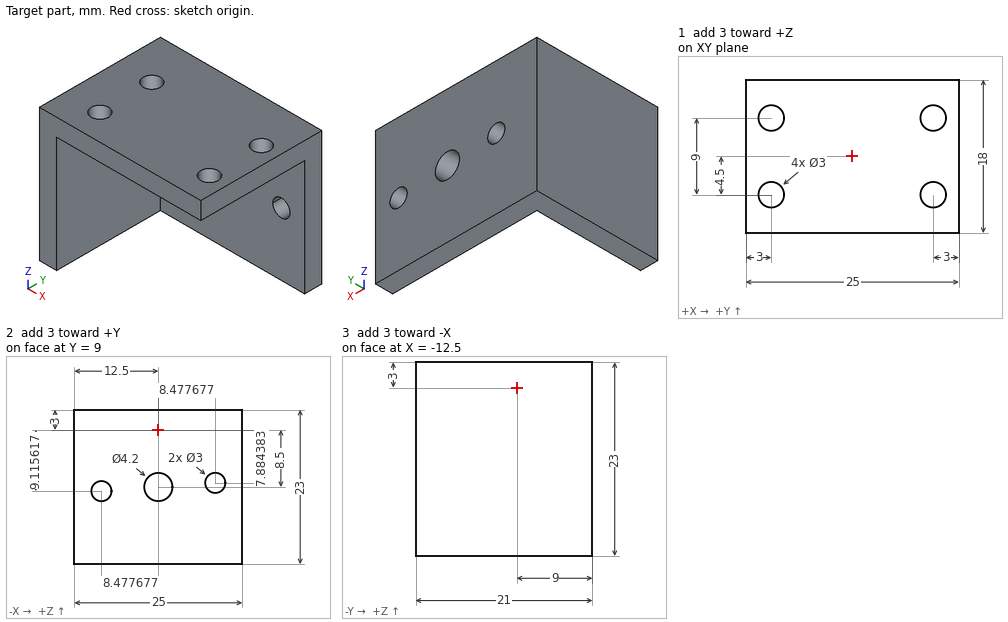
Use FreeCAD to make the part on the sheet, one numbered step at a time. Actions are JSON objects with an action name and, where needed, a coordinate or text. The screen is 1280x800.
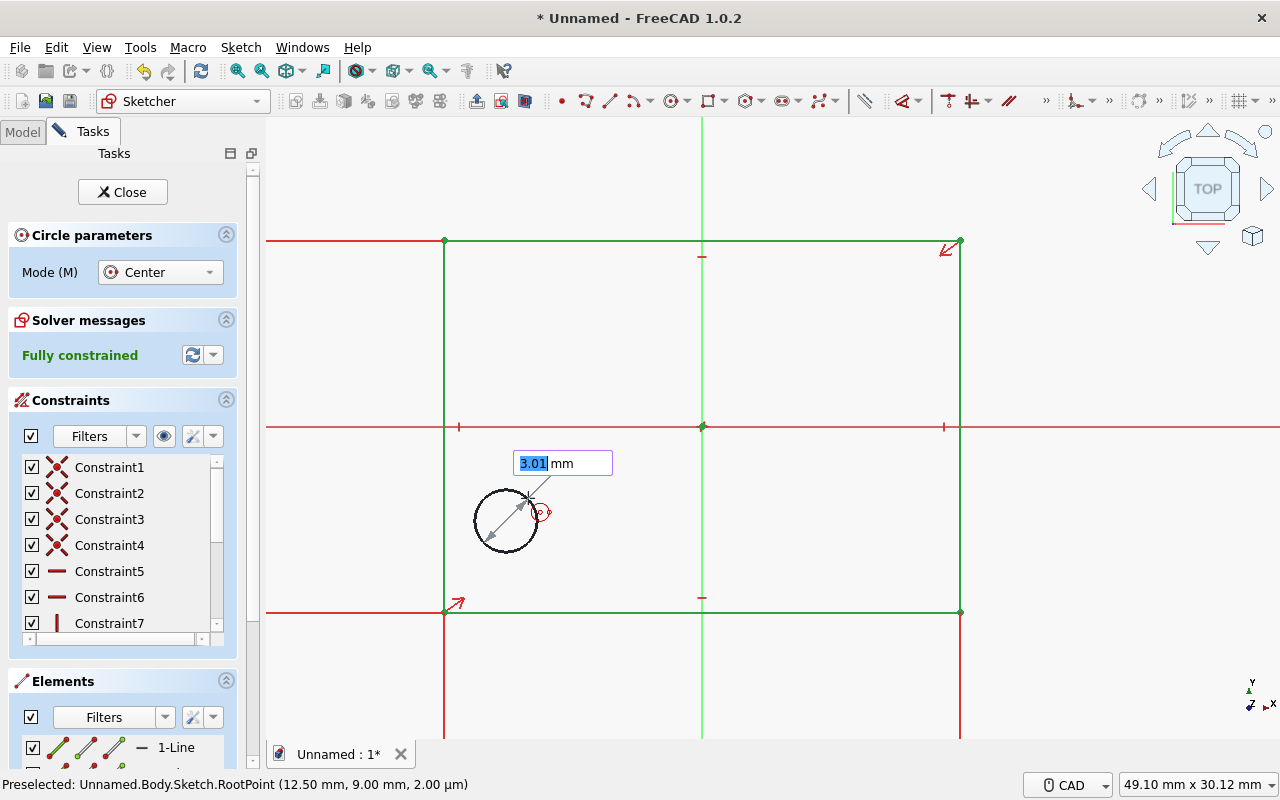
{"action": "type", "text": "3"}
{"action": "key", "text": "Return"}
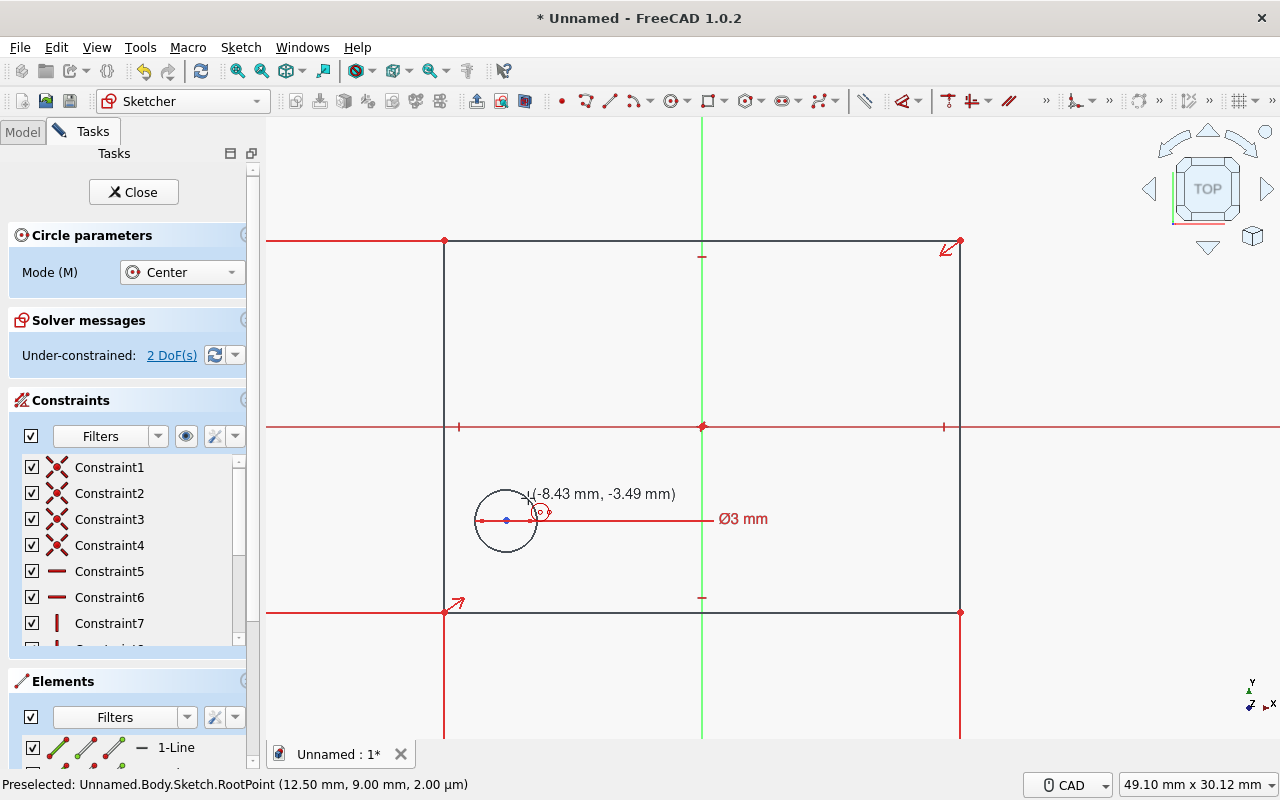
{"action": "left_click", "coordinate": [898, 520]}
{"action": "mouse_move", "coordinate": [920, 498]}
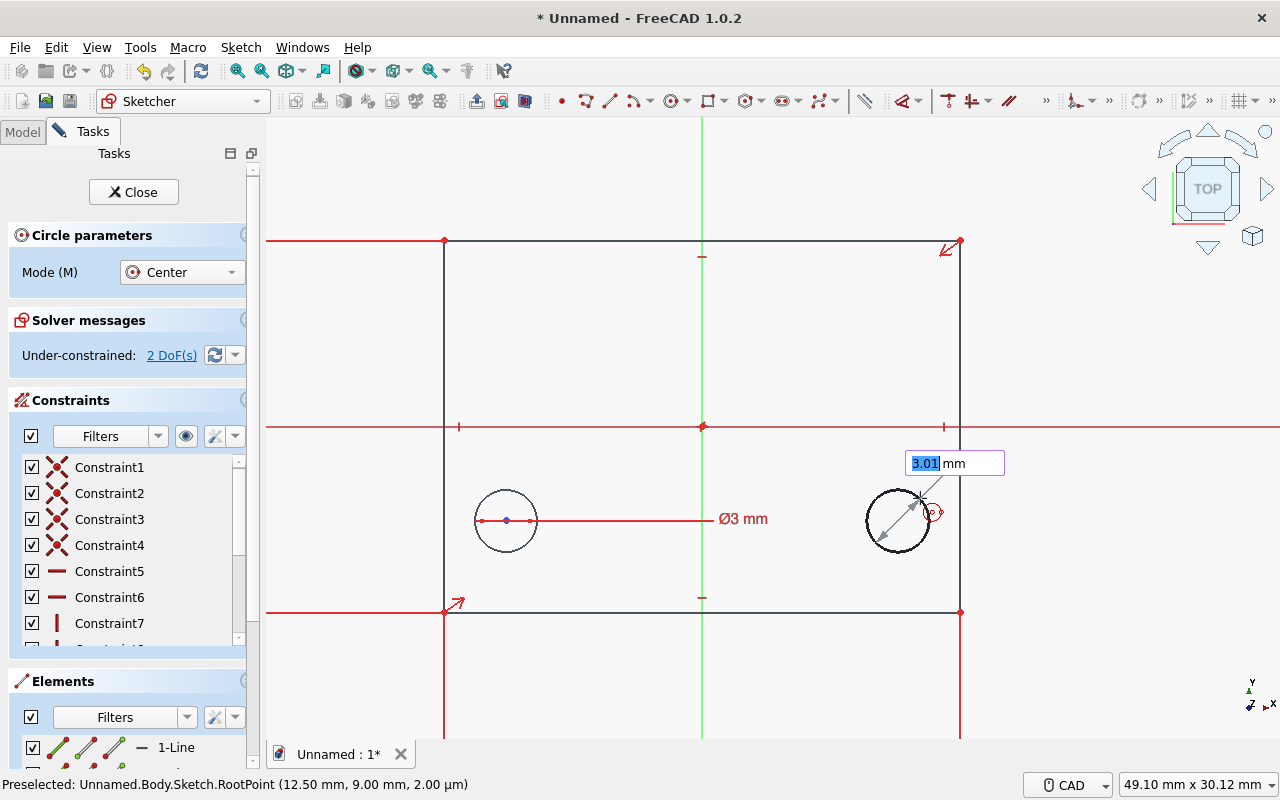
{"action": "type", "text": "3"}
{"action": "key", "text": "Return"}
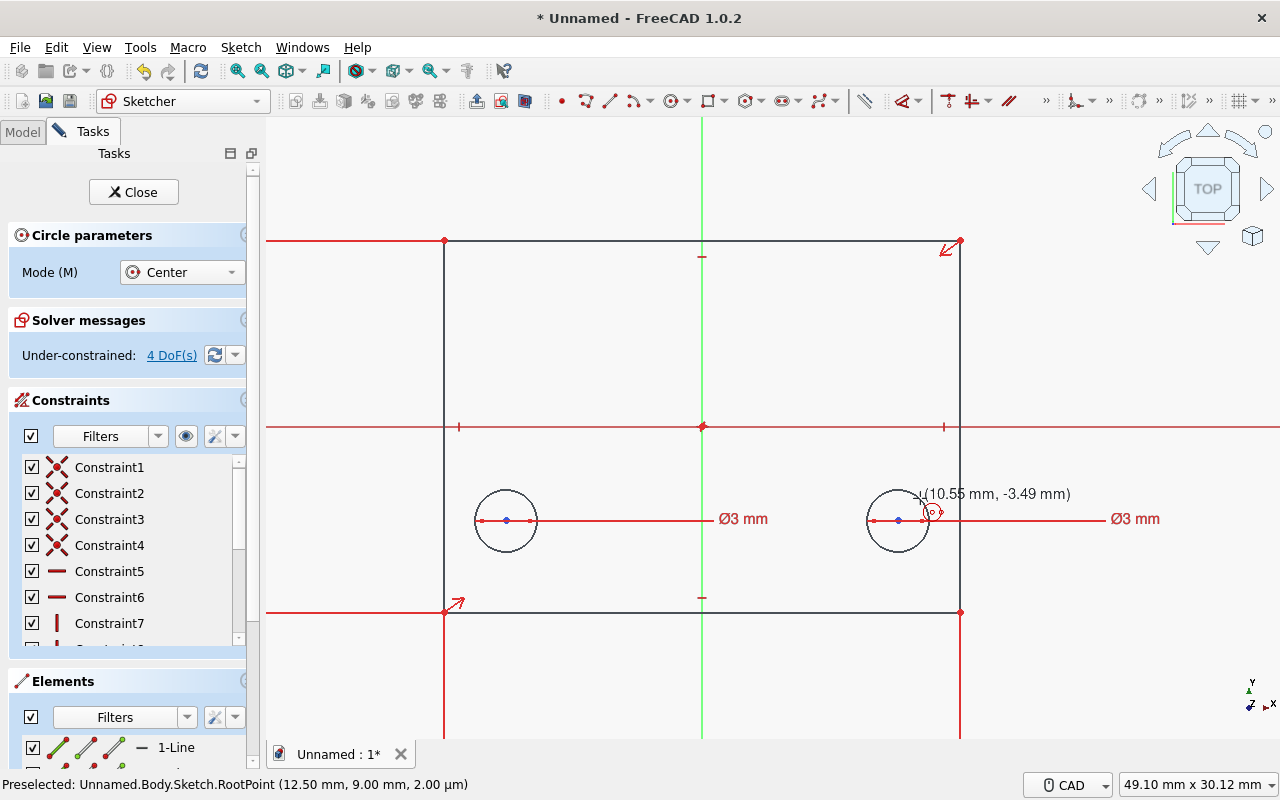
{"action": "left_click", "coordinate": [506, 334]}
{"action": "mouse_move", "coordinate": [528, 312]}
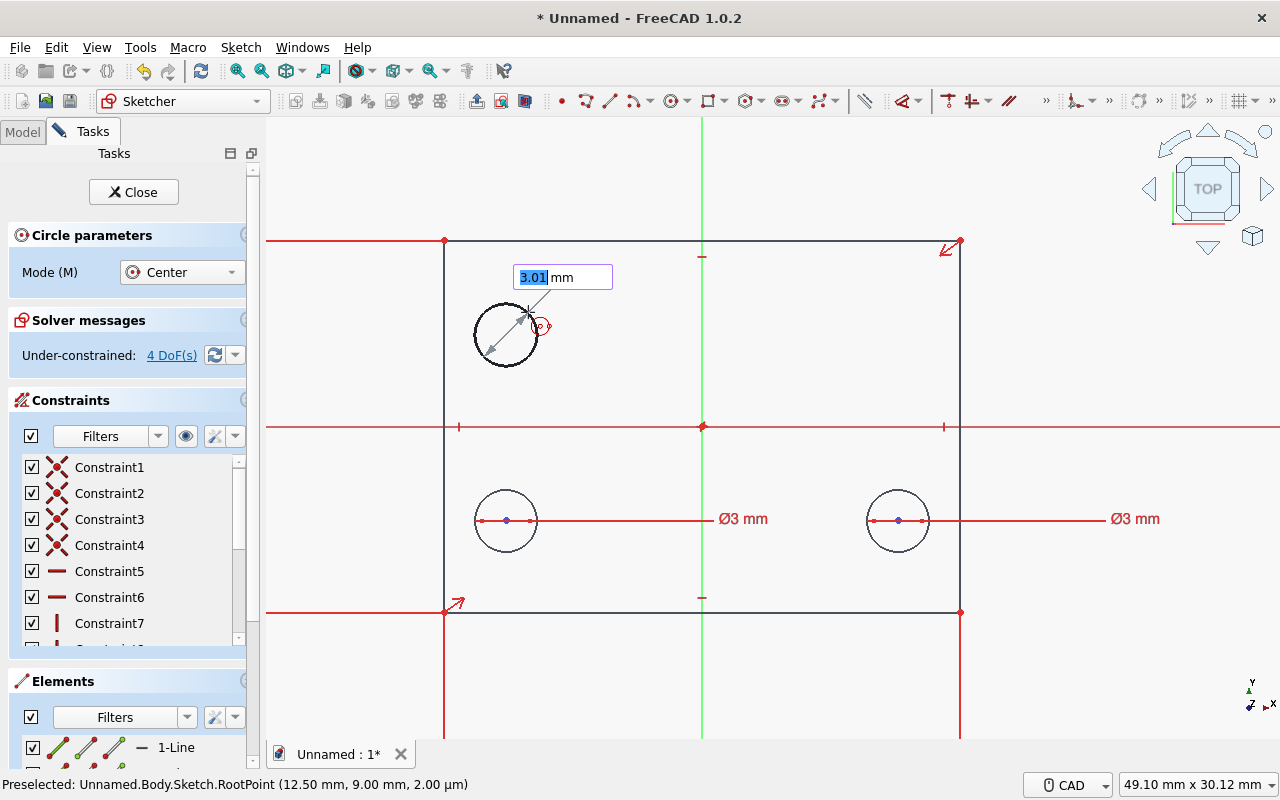
{"action": "type", "text": "3"}
{"action": "key", "text": "Return"}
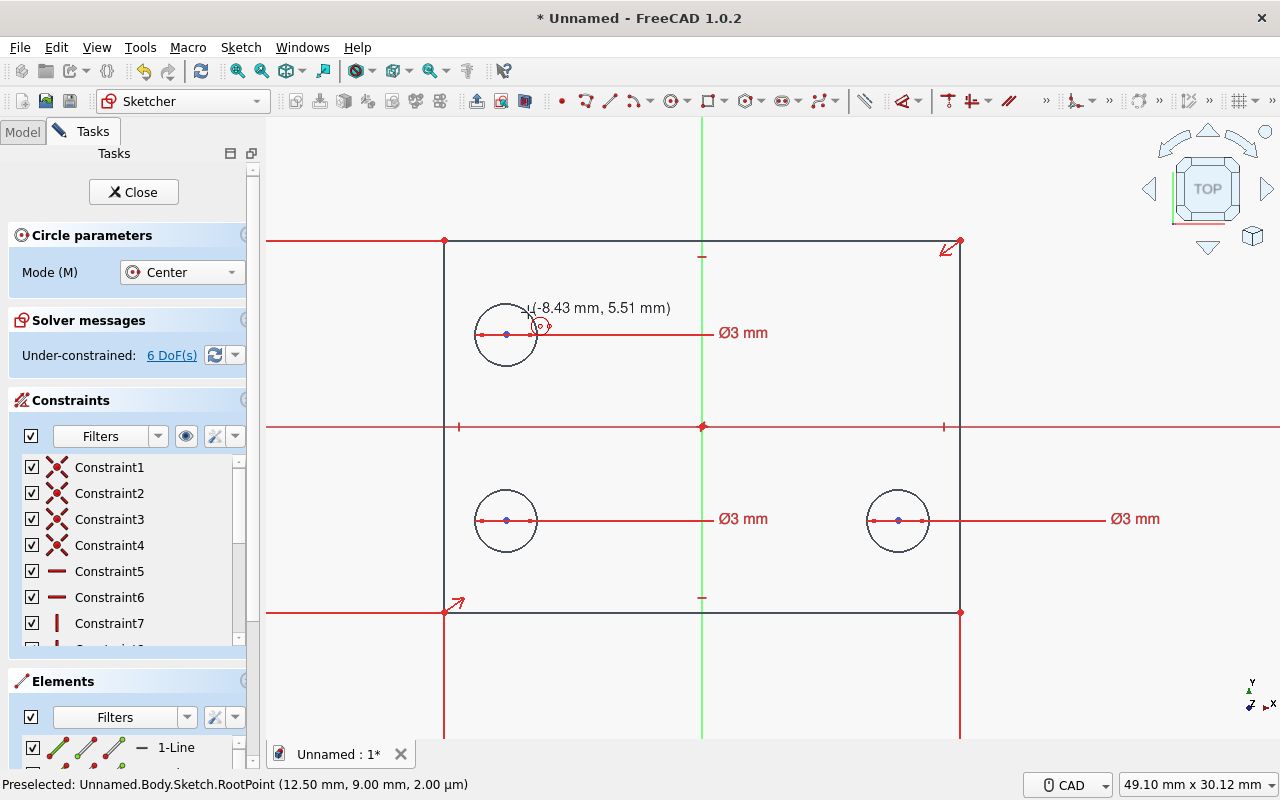
{"action": "left_click", "coordinate": [898, 334]}
{"action": "mouse_move", "coordinate": [920, 312]}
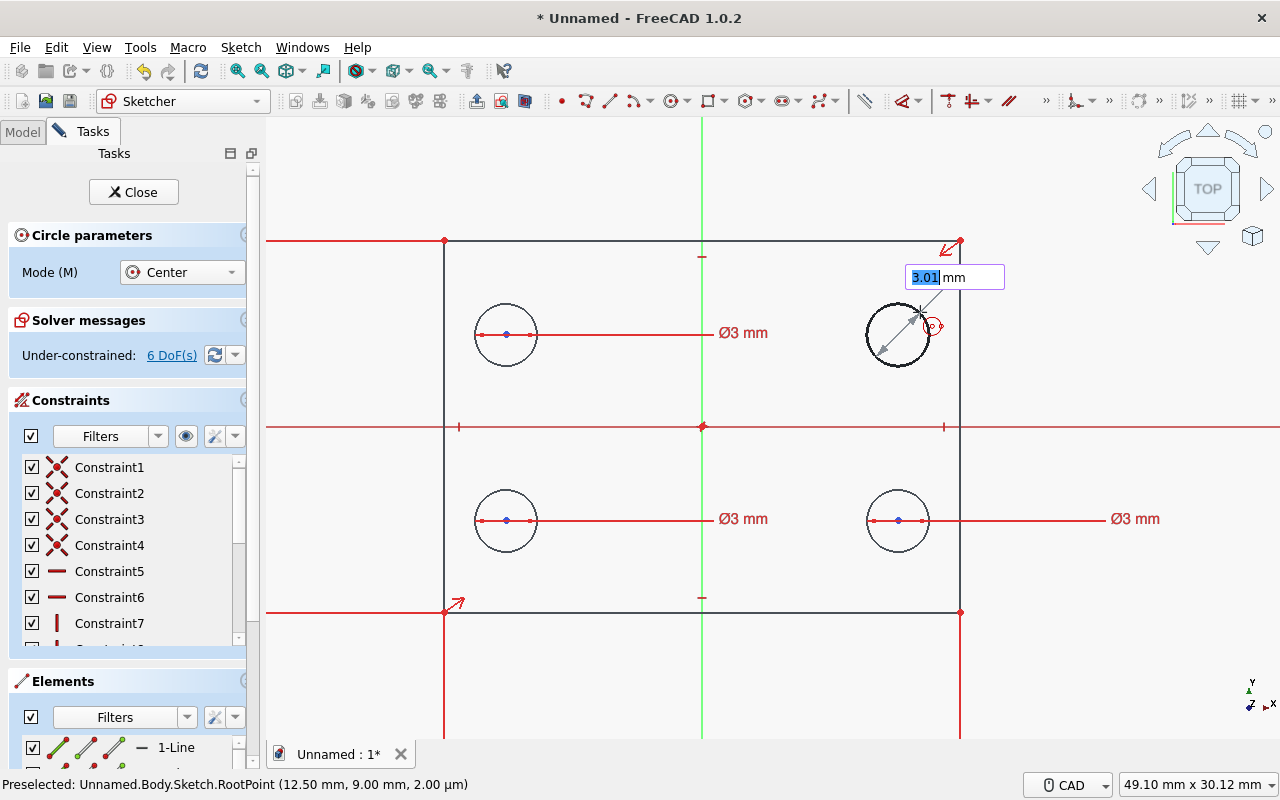
{"action": "type", "text": "3"}
{"action": "key", "text": "Return"}
{"action": "key", "text": "Escape"}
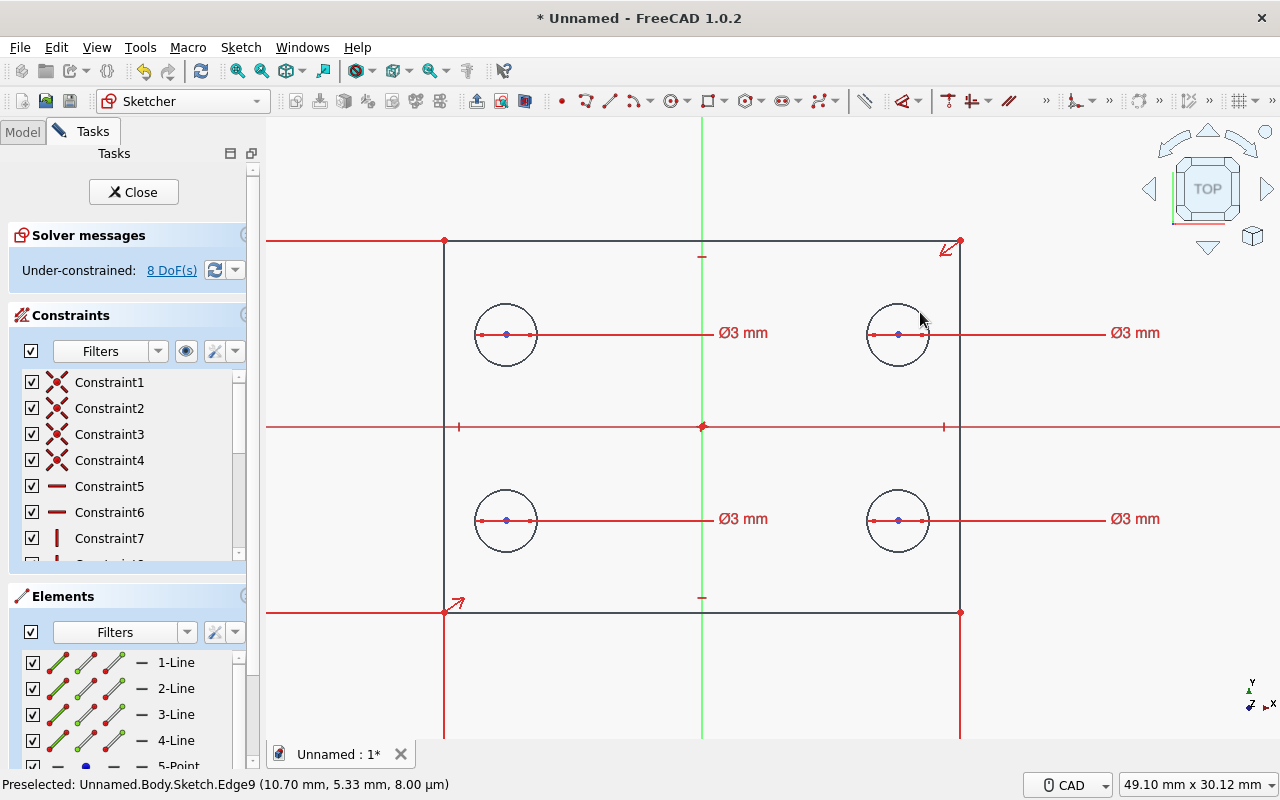
{"action": "left_click", "coordinate": [506, 521]}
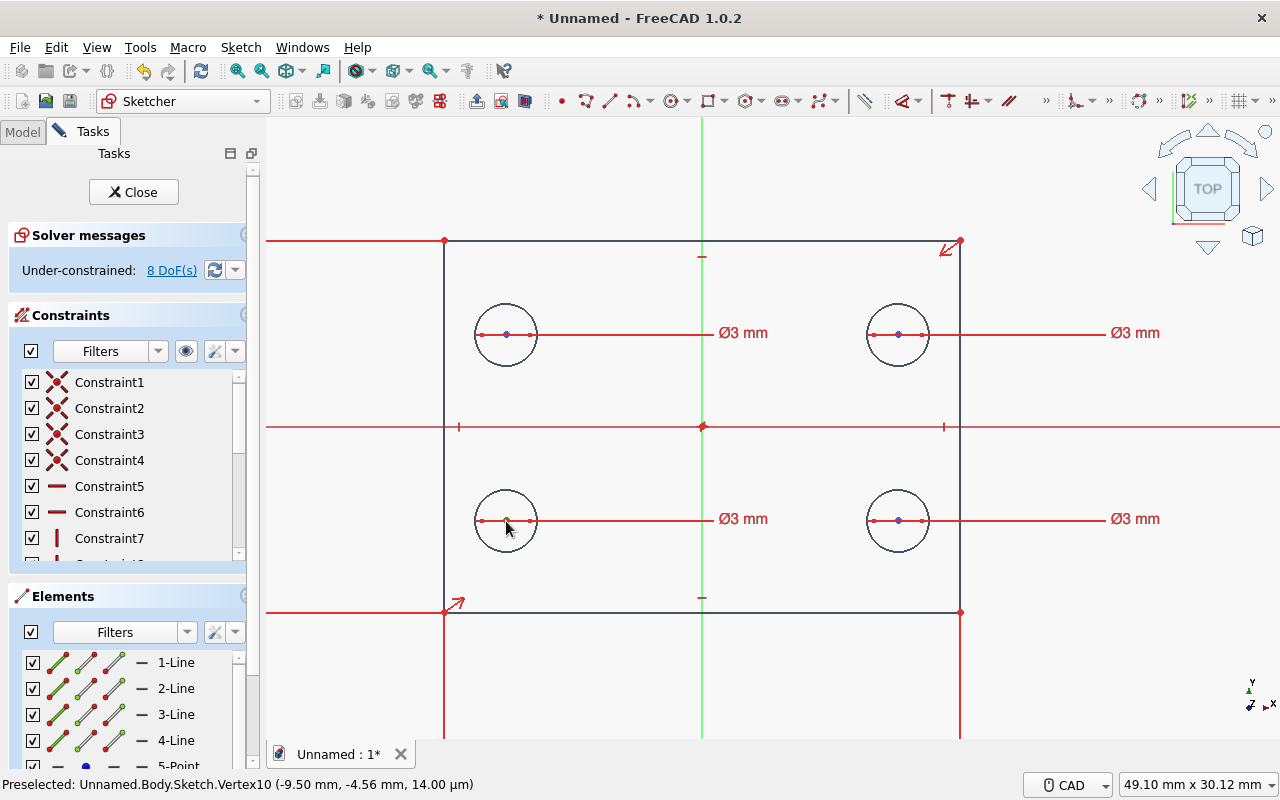
{"action": "left_click", "coordinate": [898, 521]}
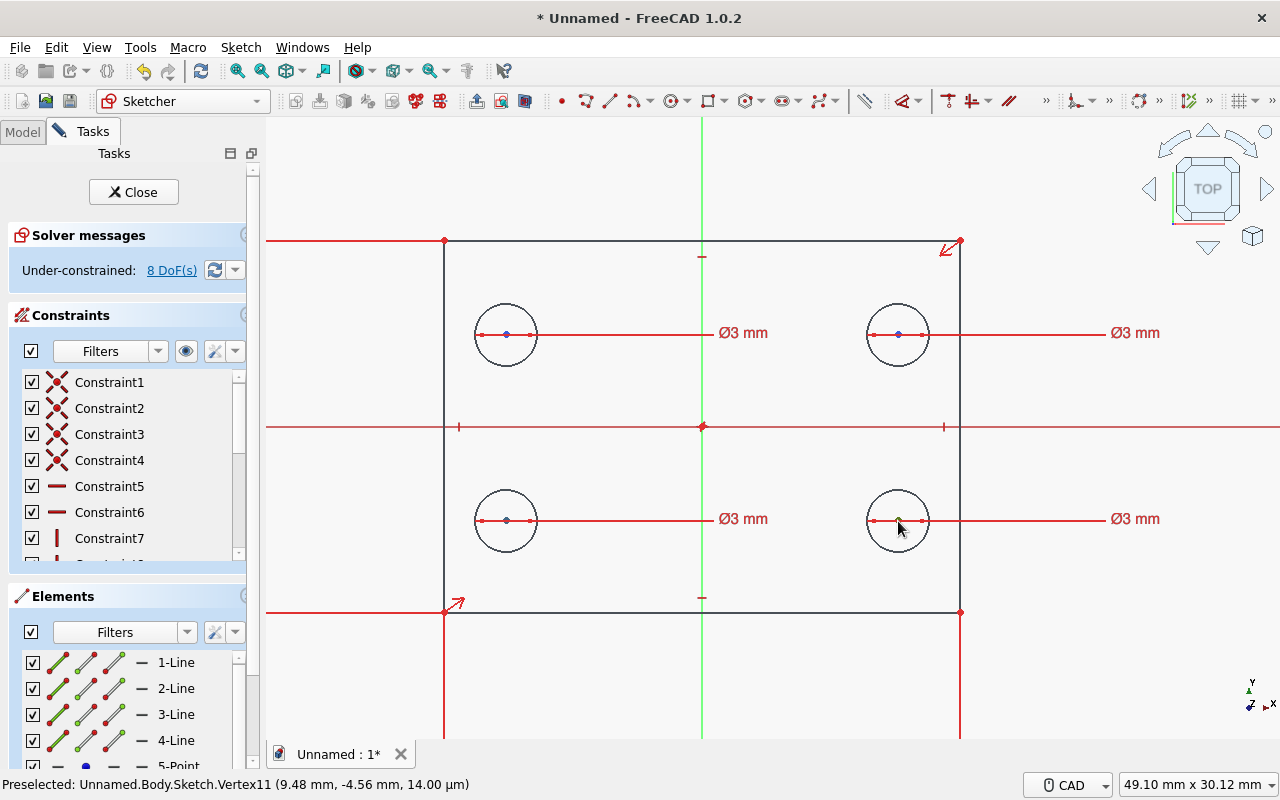
{"action": "key", "text": "h"}